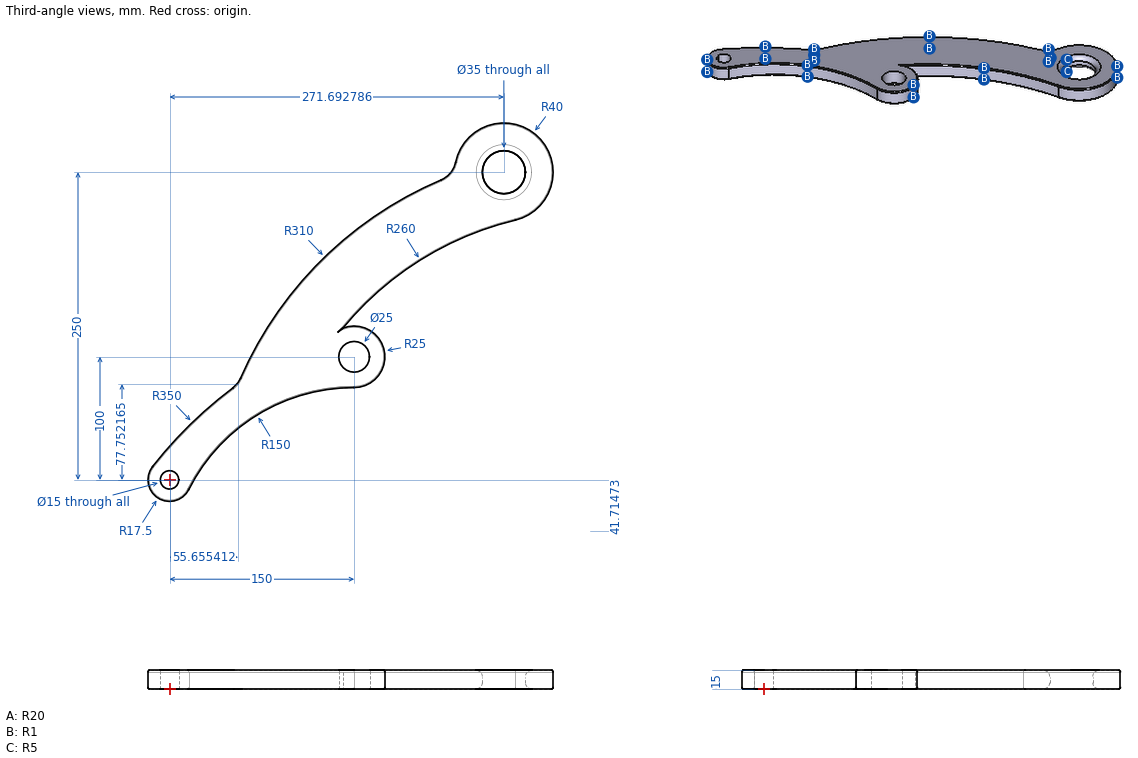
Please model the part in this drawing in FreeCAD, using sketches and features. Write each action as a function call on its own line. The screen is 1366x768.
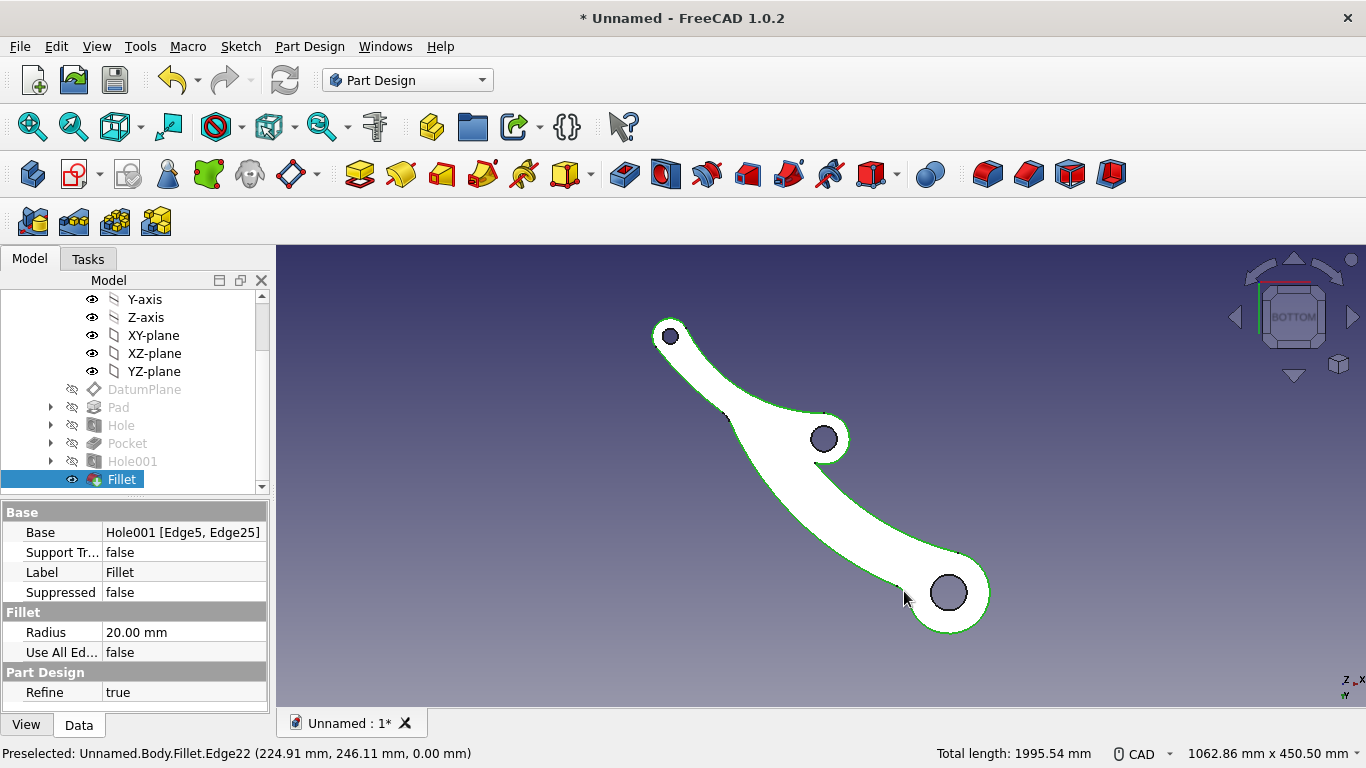
scroll(727, 415, up, 7)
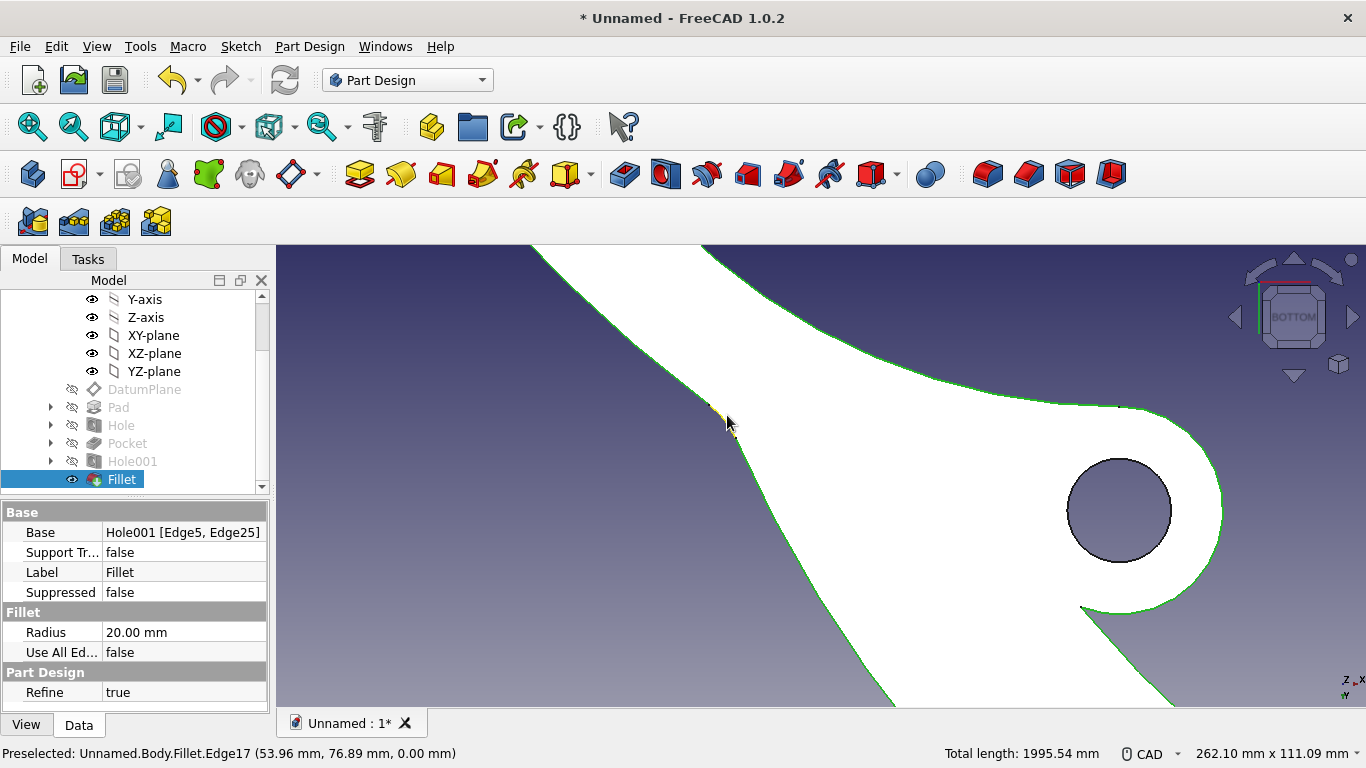
click(725, 419, ctrl)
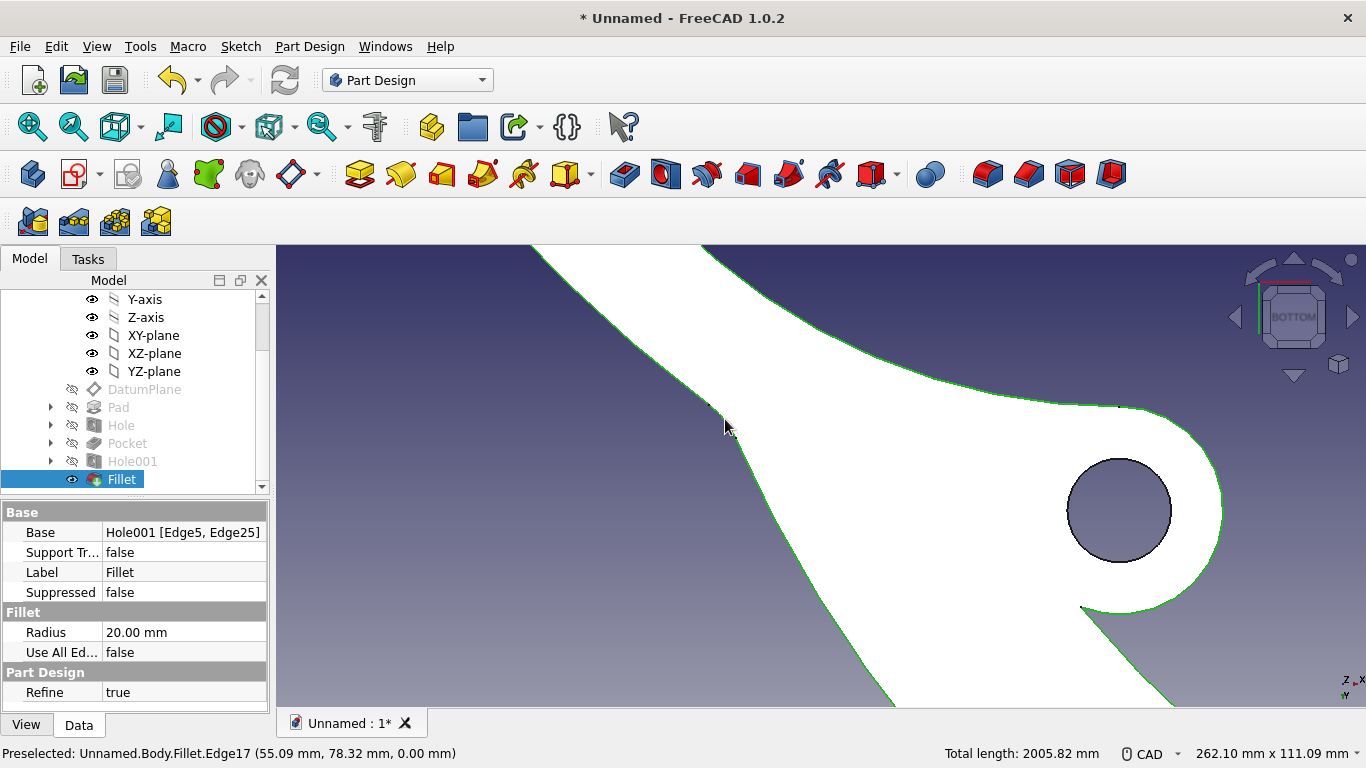
click(33, 128)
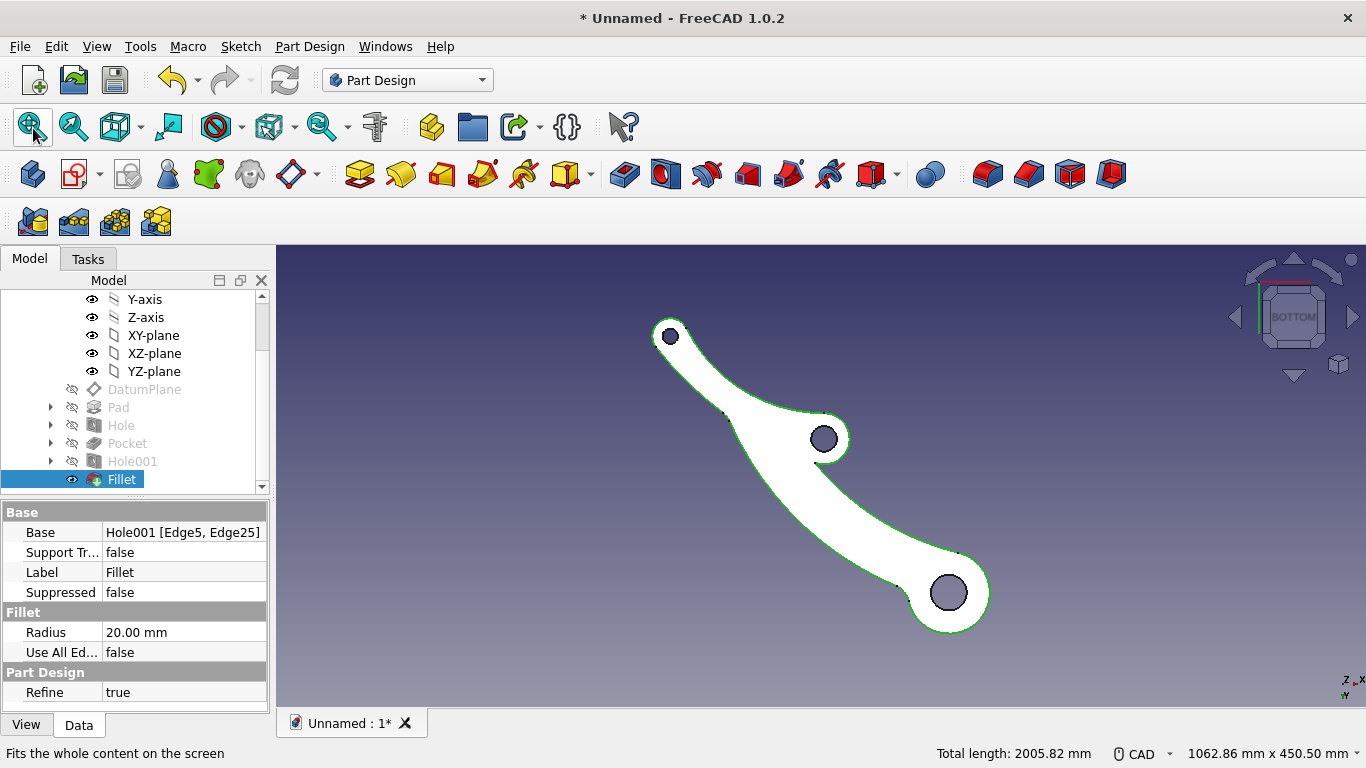
key(4)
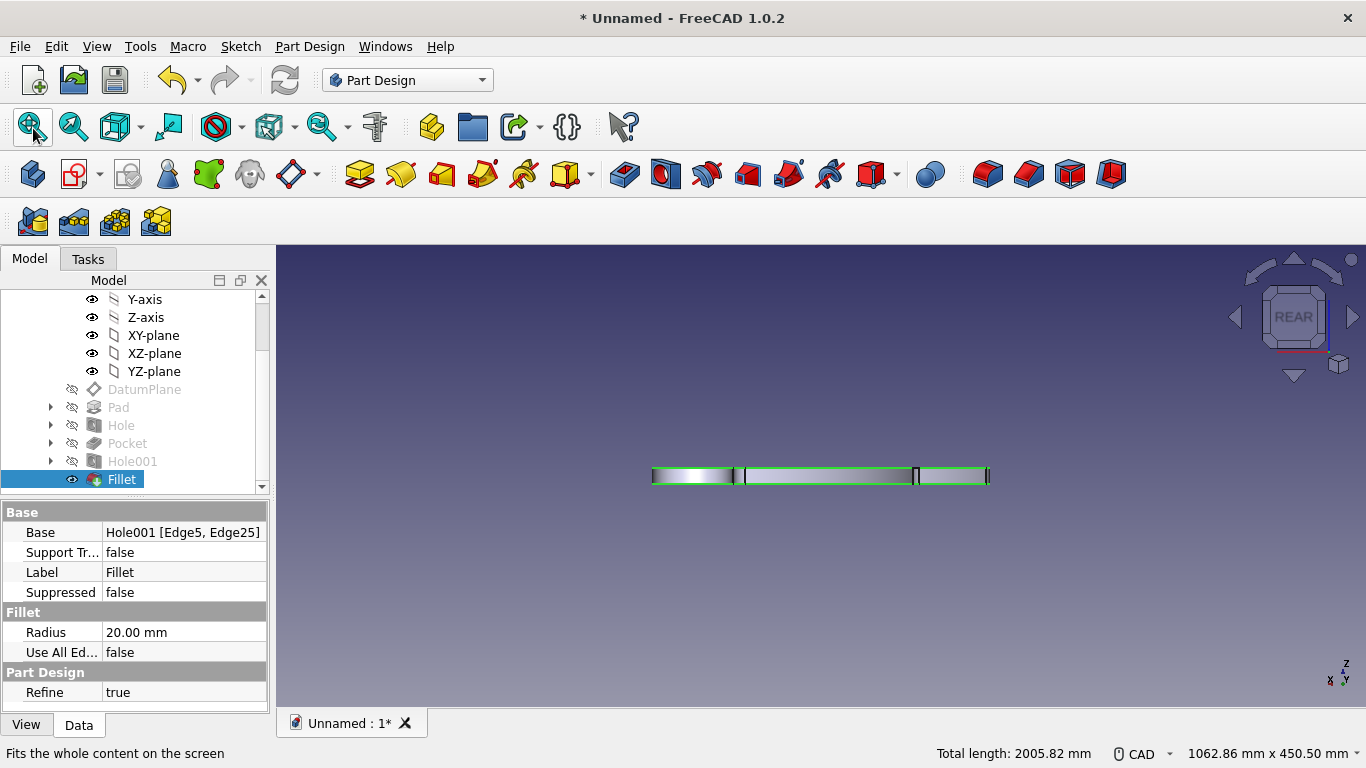
click(33, 128)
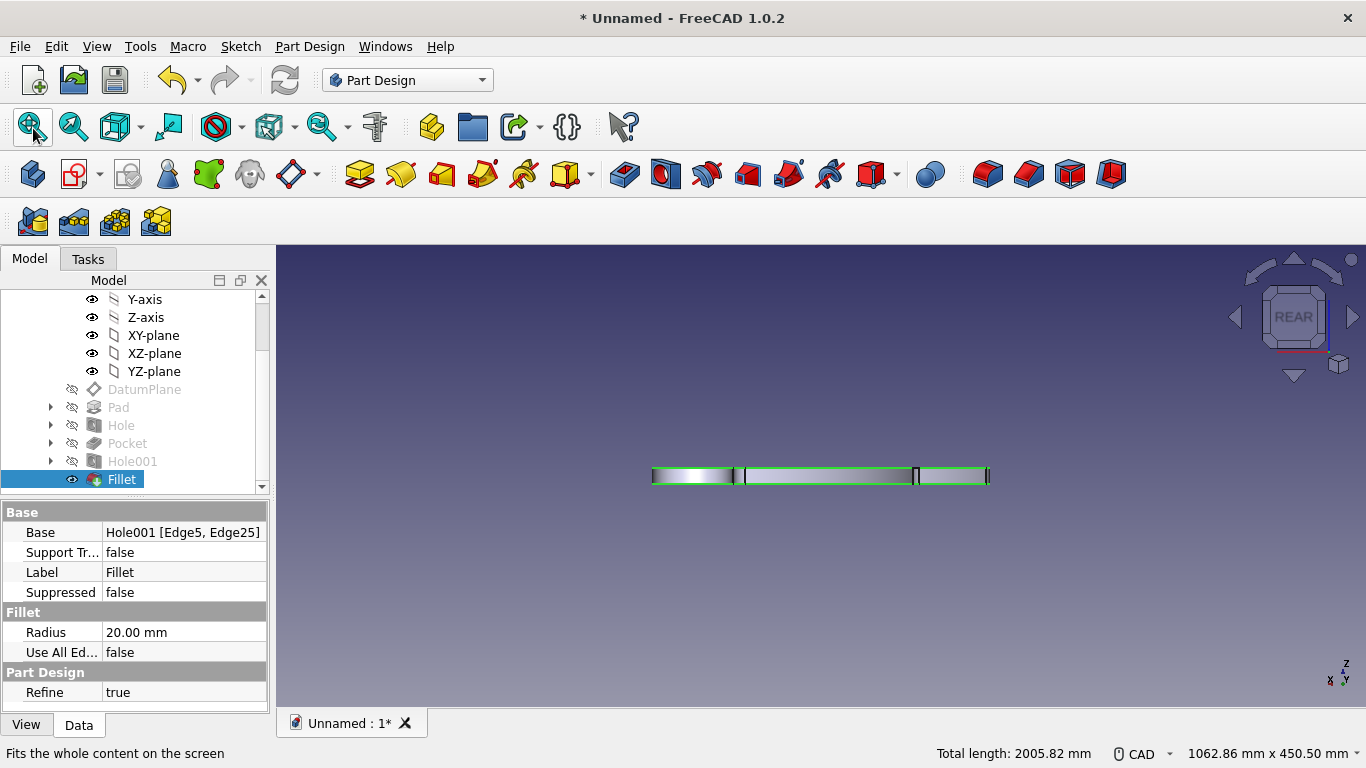
scroll(915, 467, up, 7)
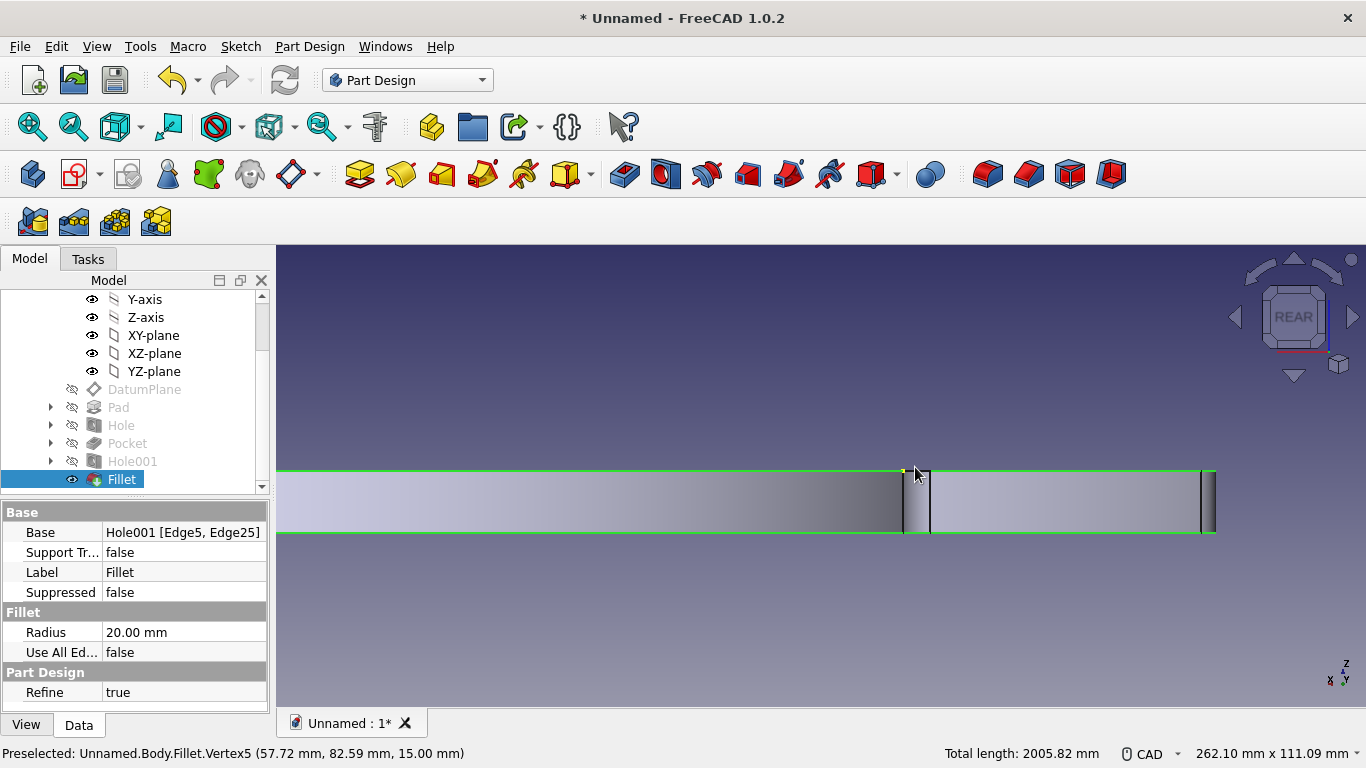
click(914, 470, ctrl)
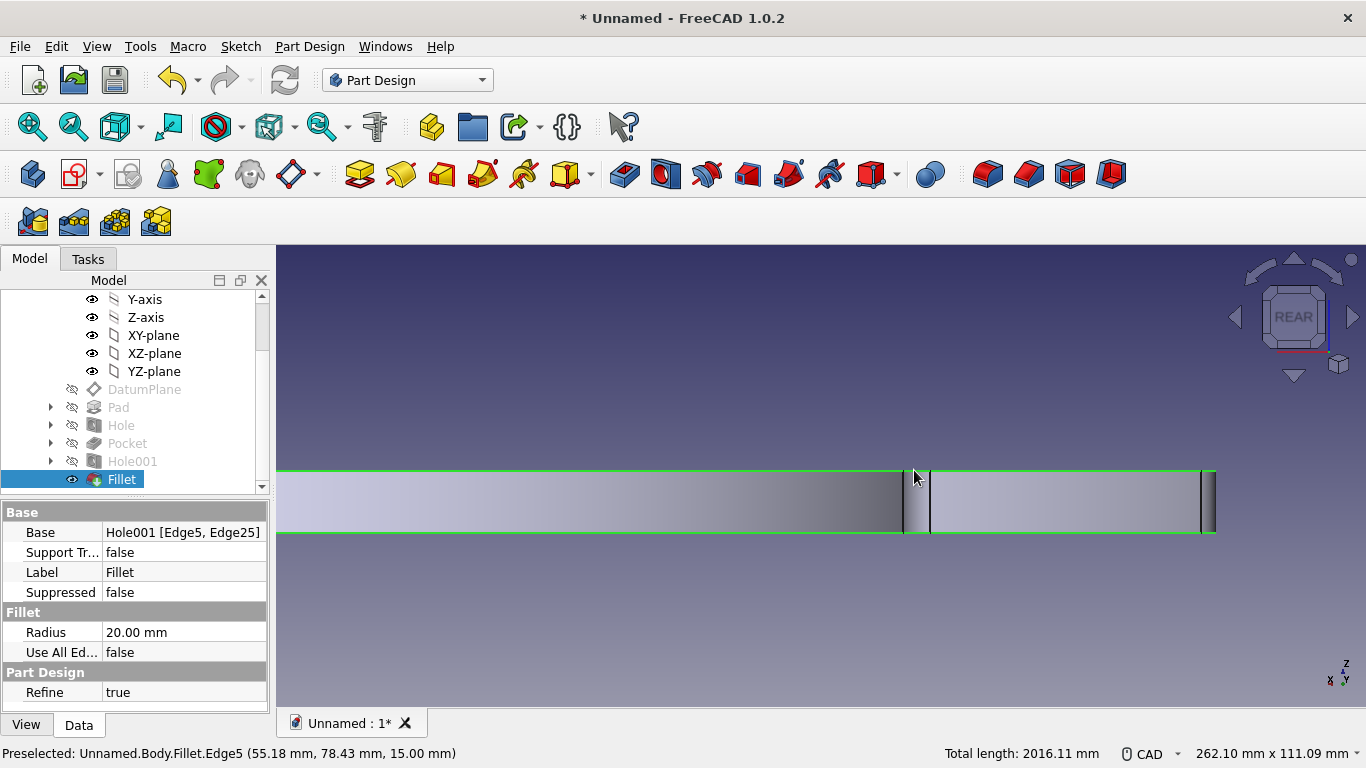
click(988, 174)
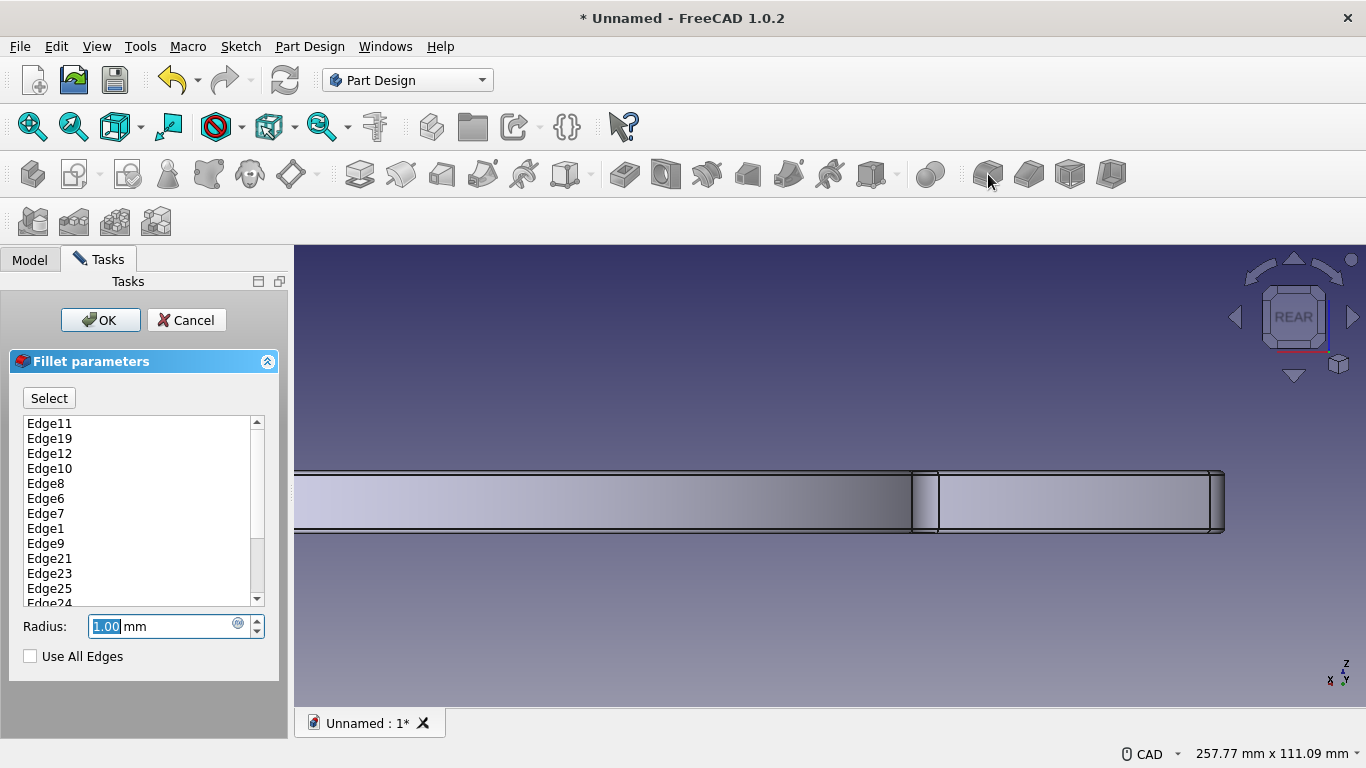
text(1)
key(Tab)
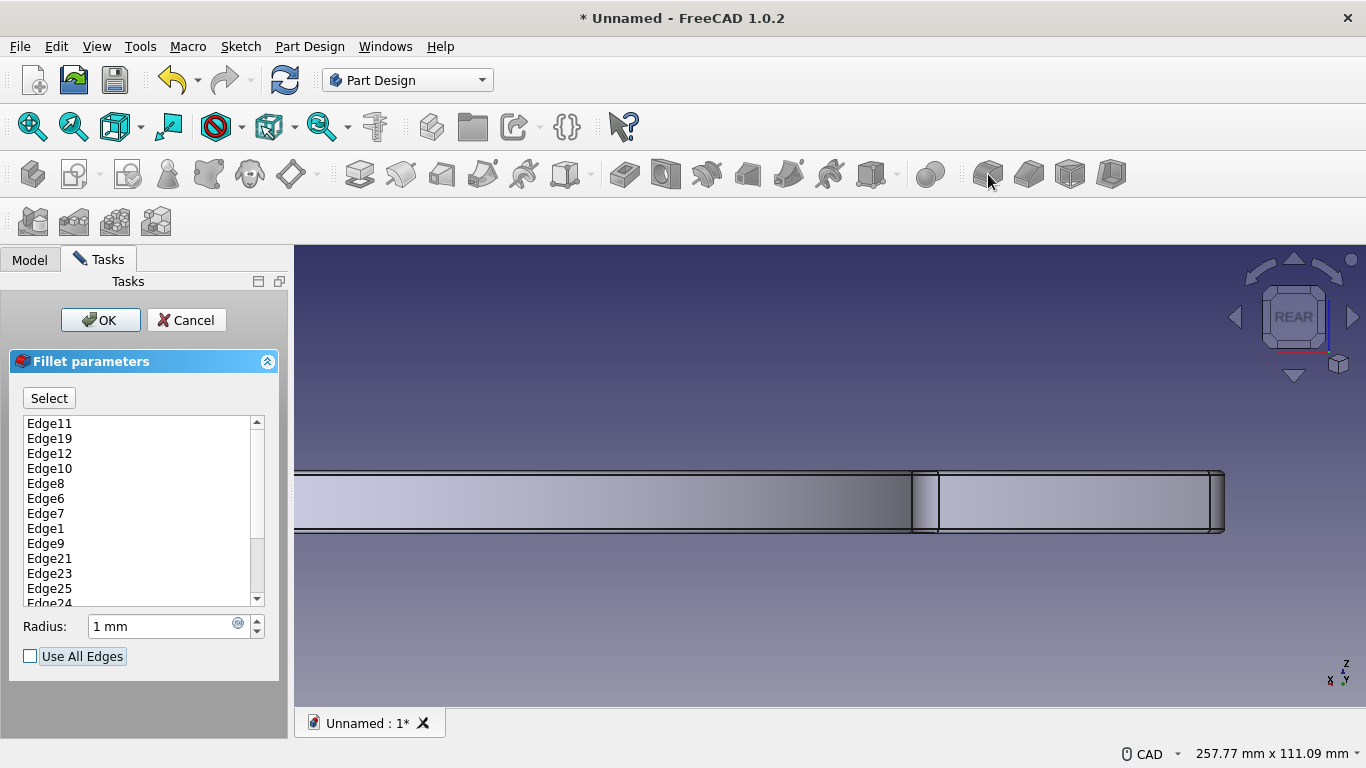
click(101, 320)